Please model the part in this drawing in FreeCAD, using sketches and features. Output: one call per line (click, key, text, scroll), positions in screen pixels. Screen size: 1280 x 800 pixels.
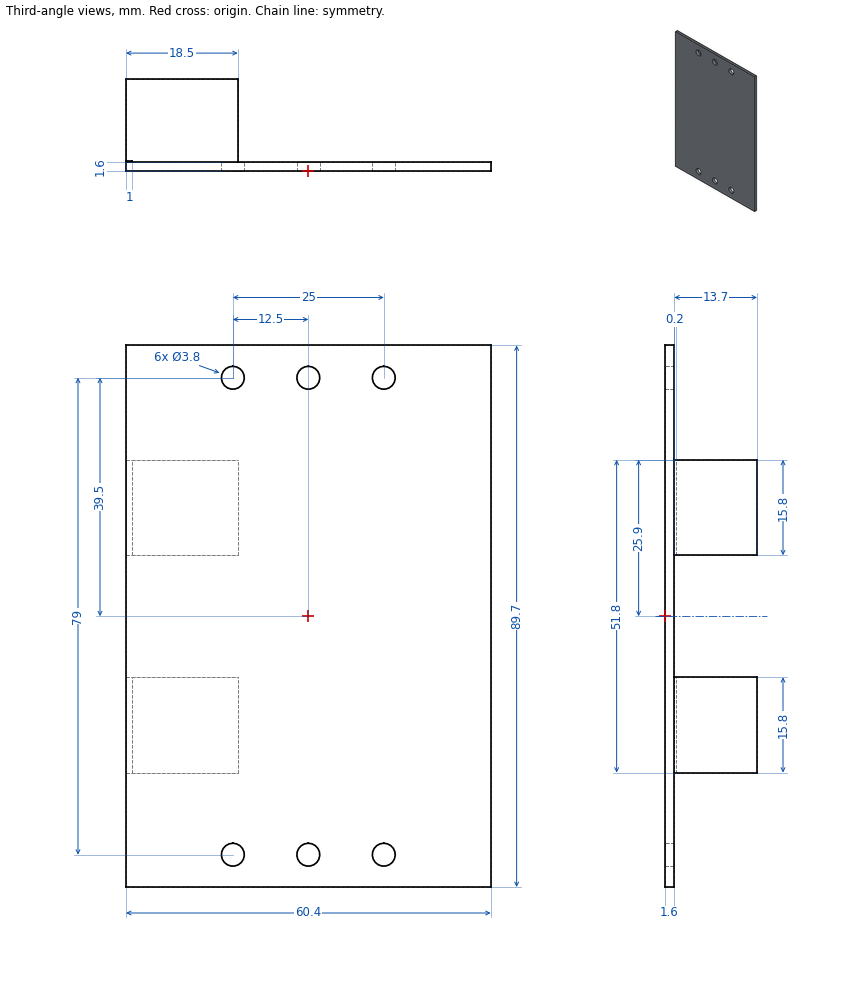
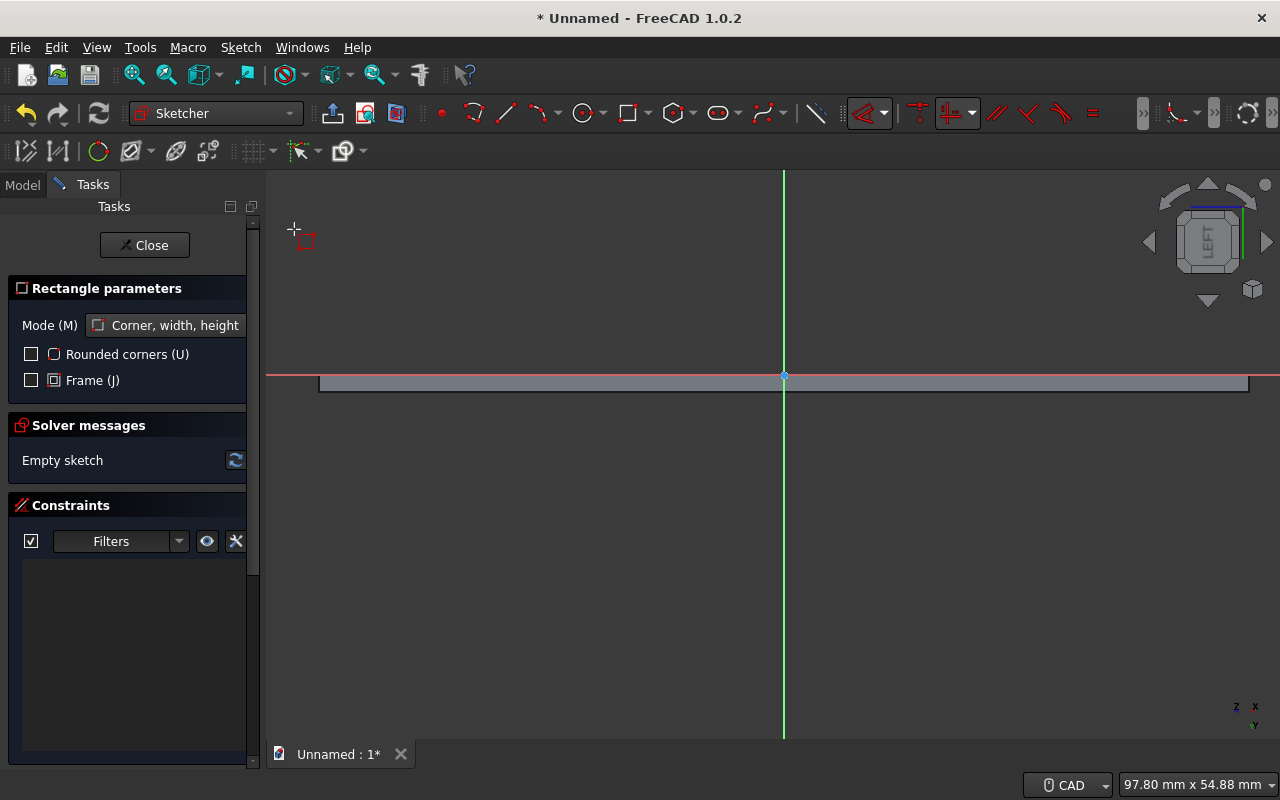
click(516, 392)
move(679, 534)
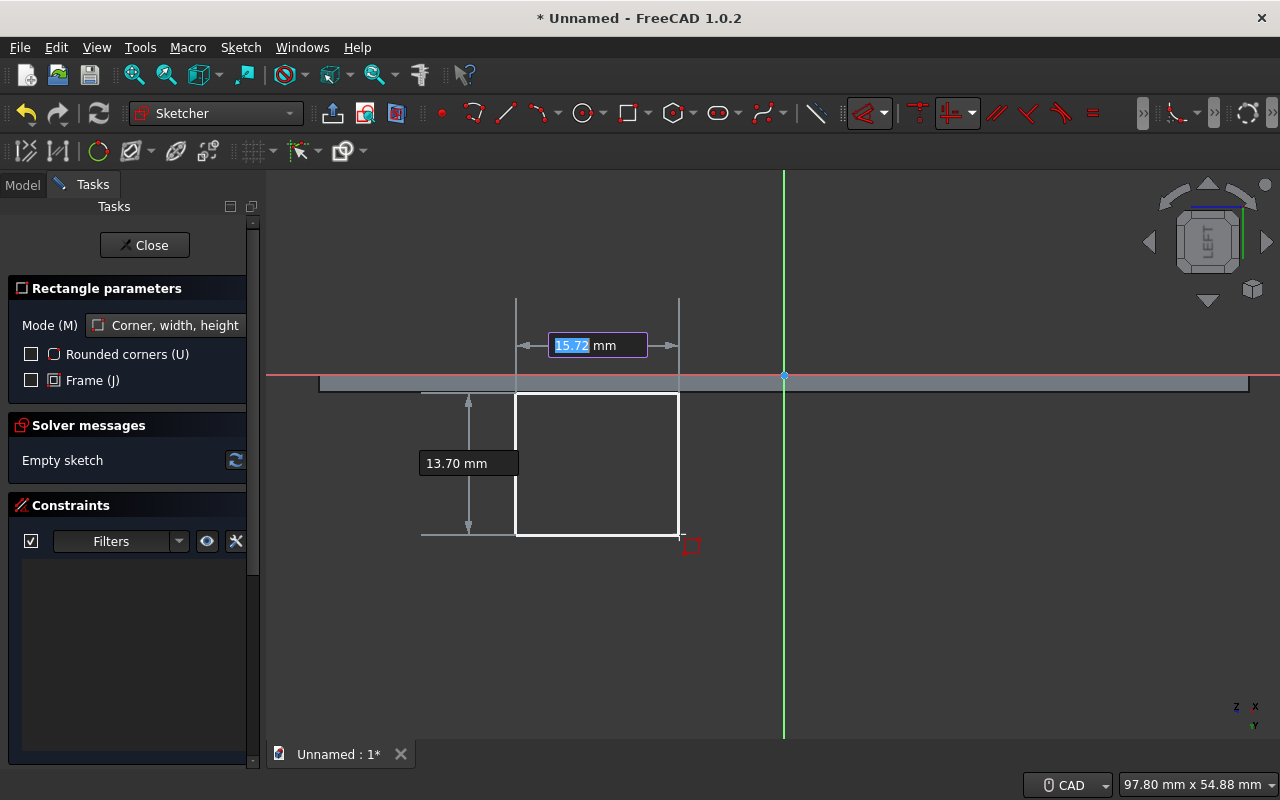
text(15.8)
key(Tab)
text(13.7)
key(Return)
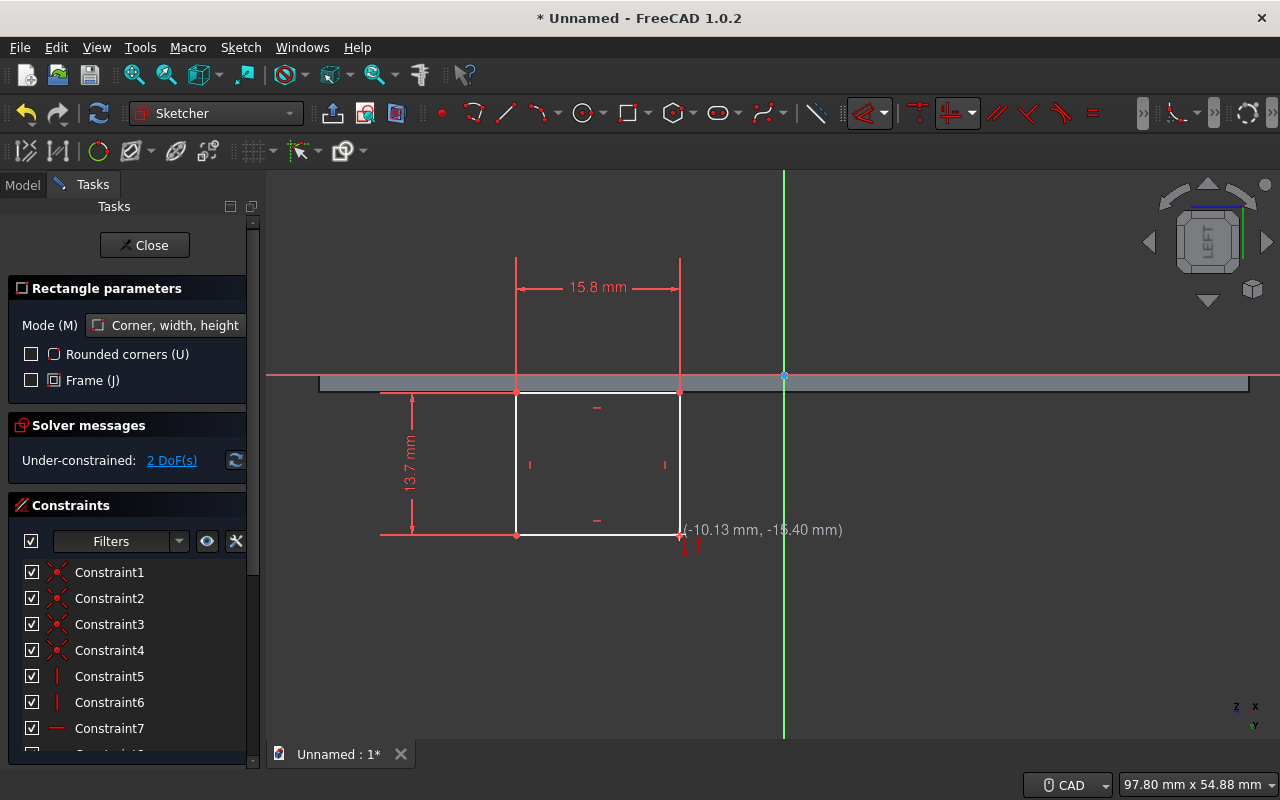
click(889, 392)
move(1053, 534)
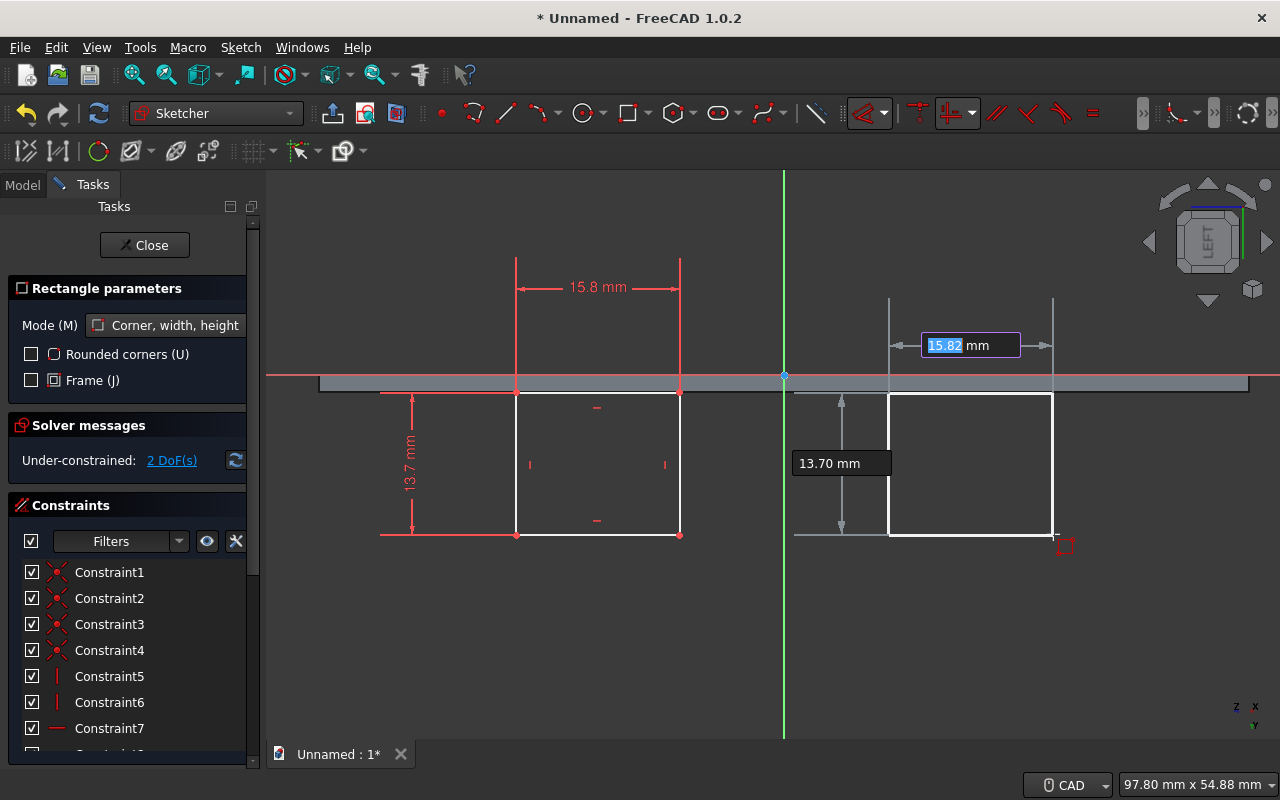
text(15.8)
key(Tab)
text(13.7)
key(Return)
key(Escape)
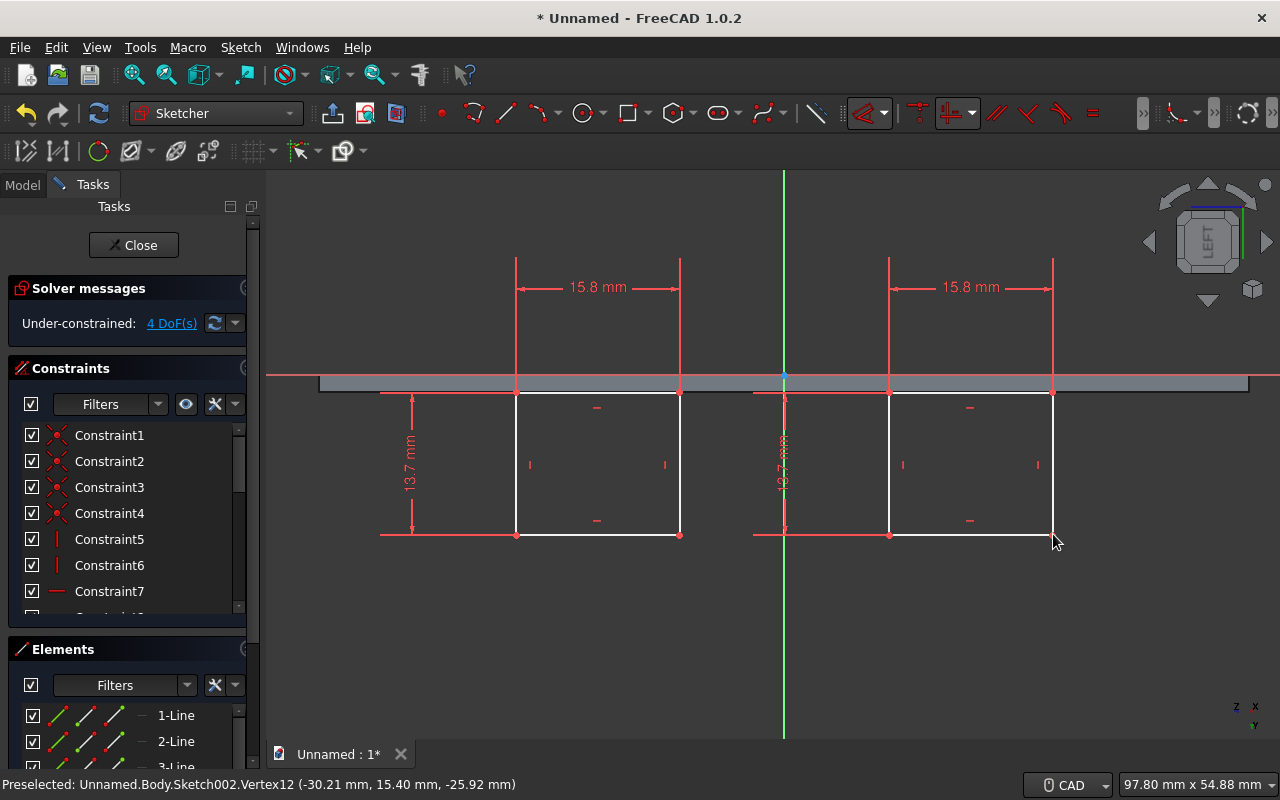
click(680, 393)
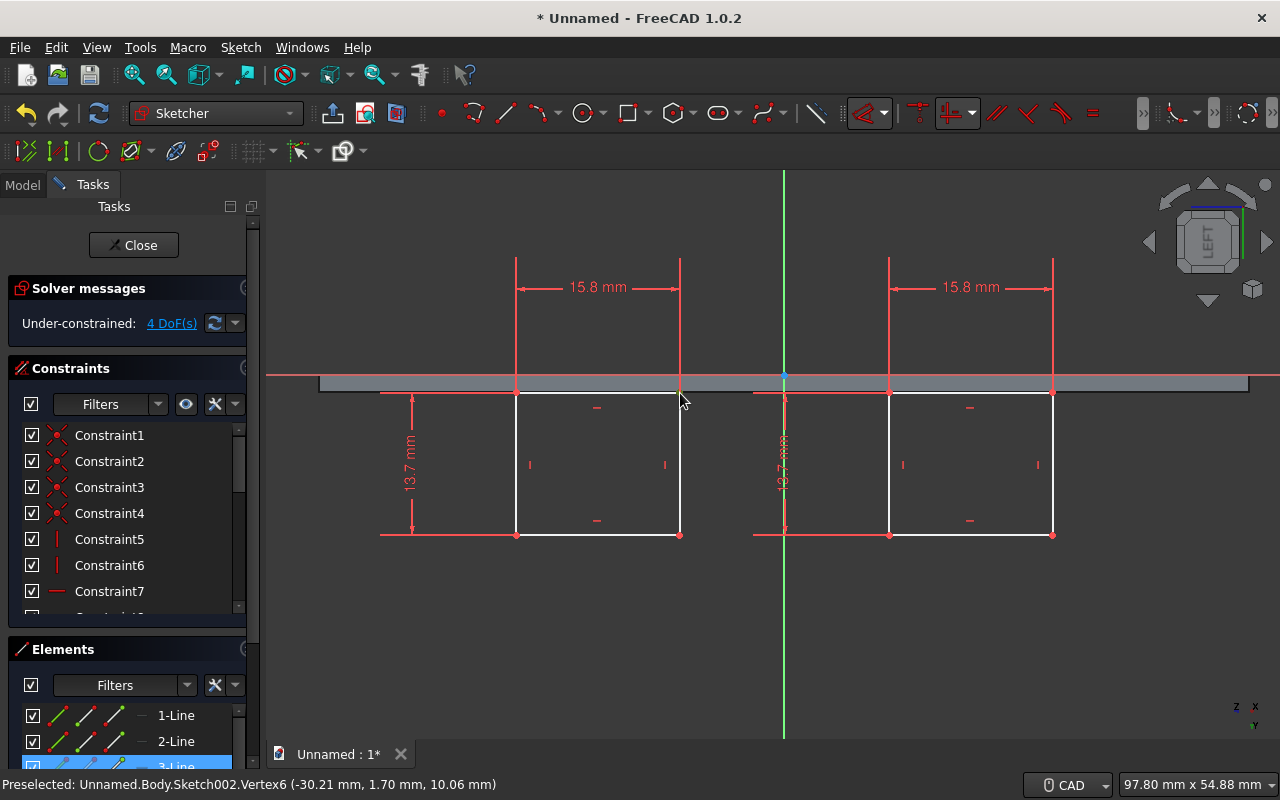
click(889, 393)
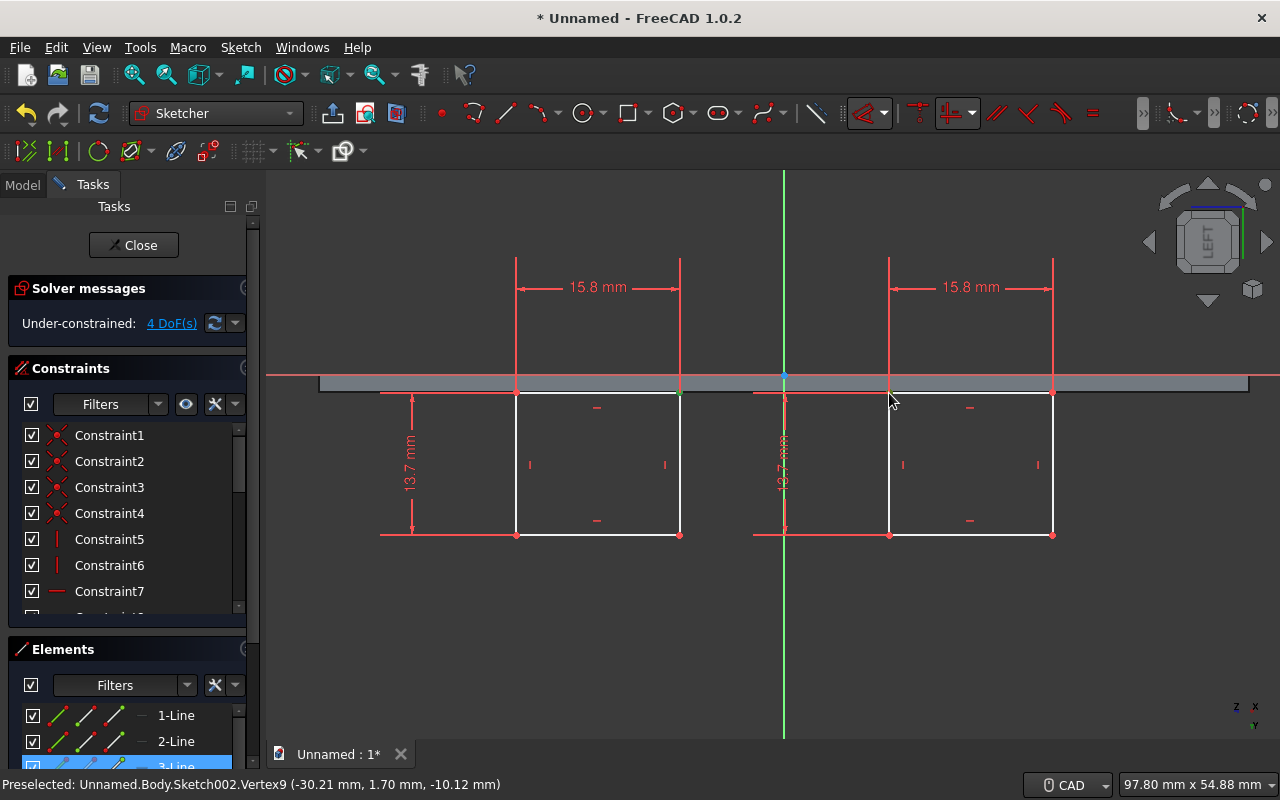
click(784, 674)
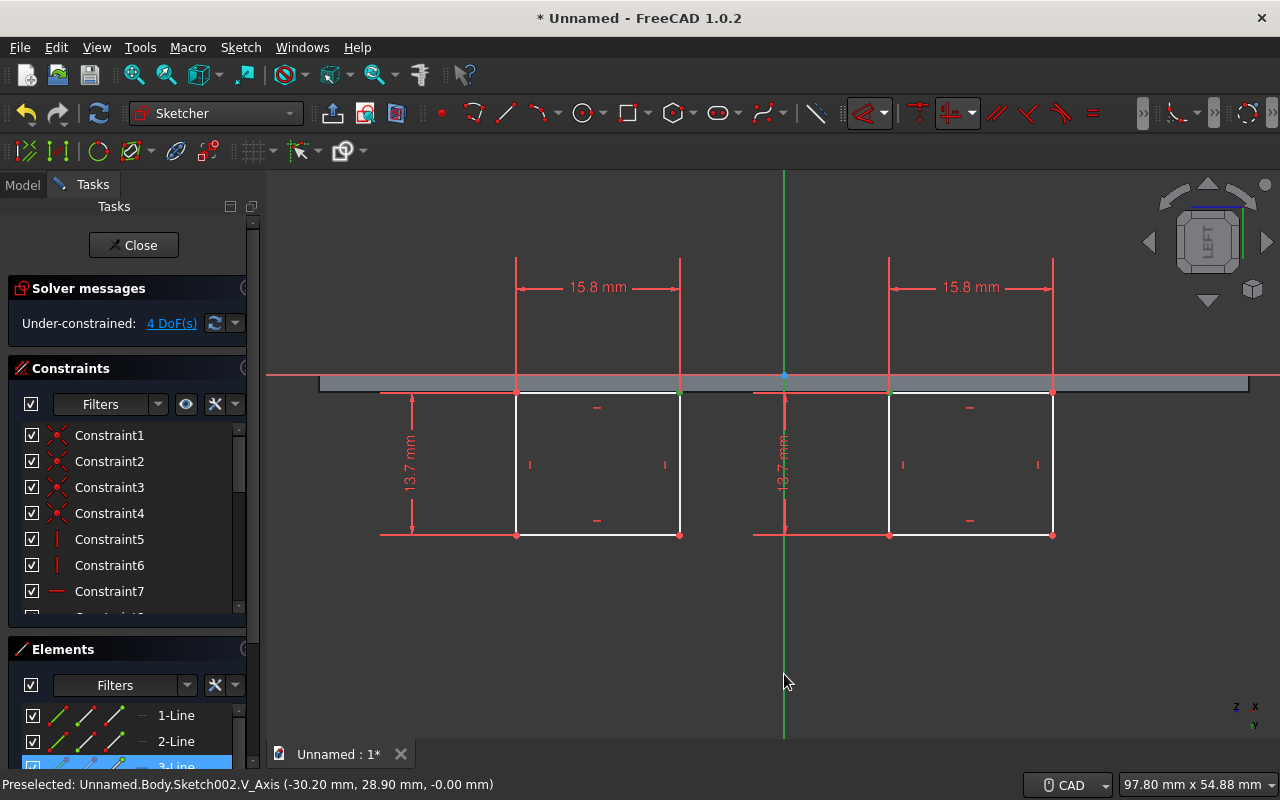
key(s)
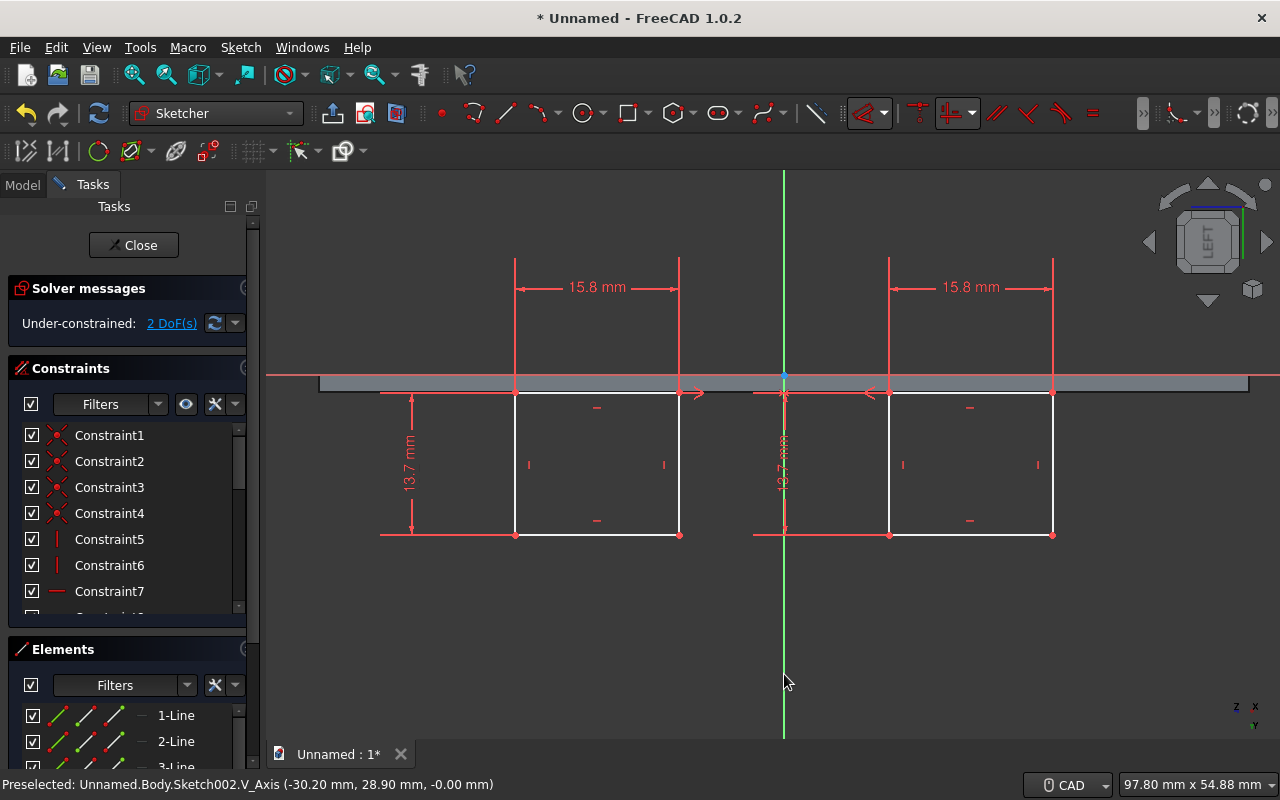
scroll(515, 393, up, 5)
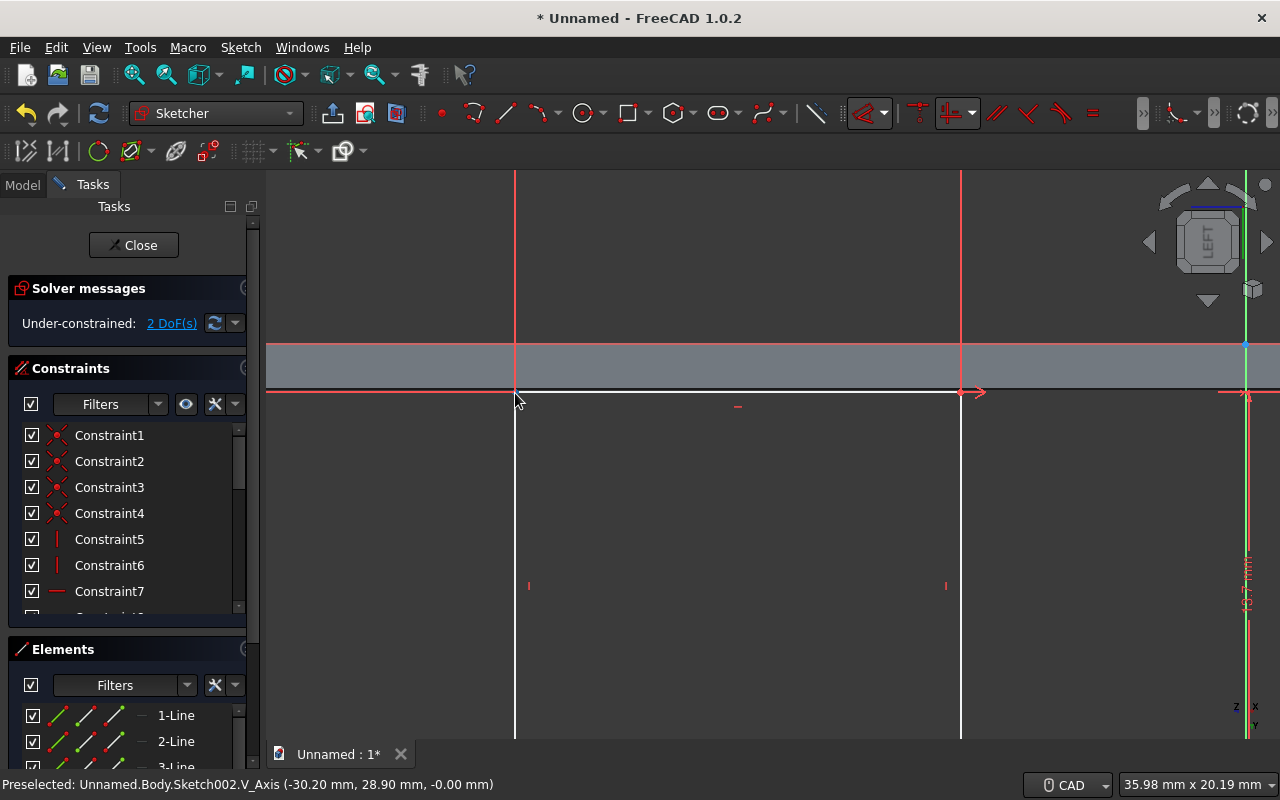
click(515, 392)